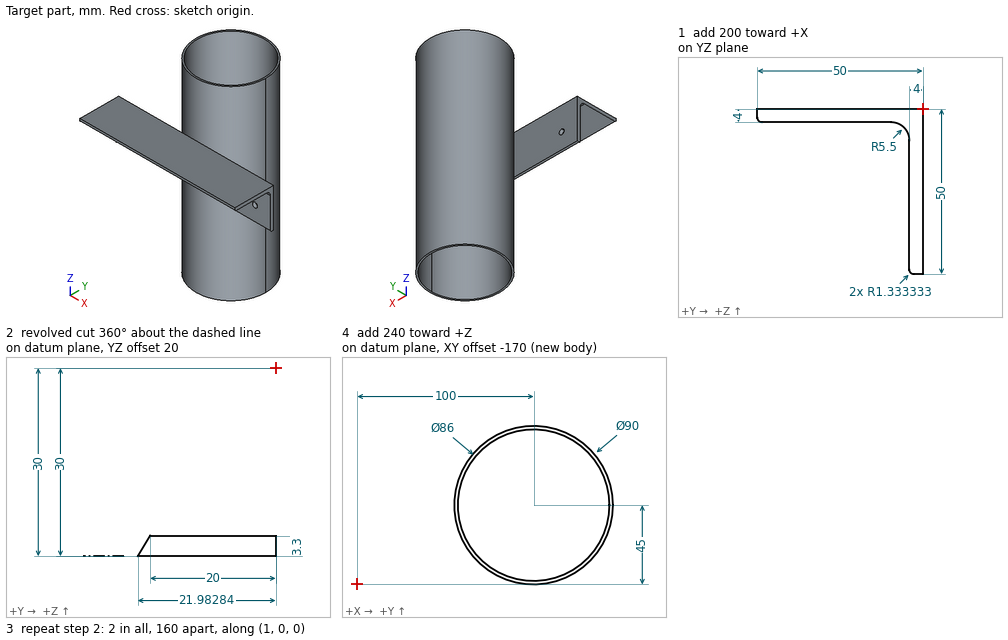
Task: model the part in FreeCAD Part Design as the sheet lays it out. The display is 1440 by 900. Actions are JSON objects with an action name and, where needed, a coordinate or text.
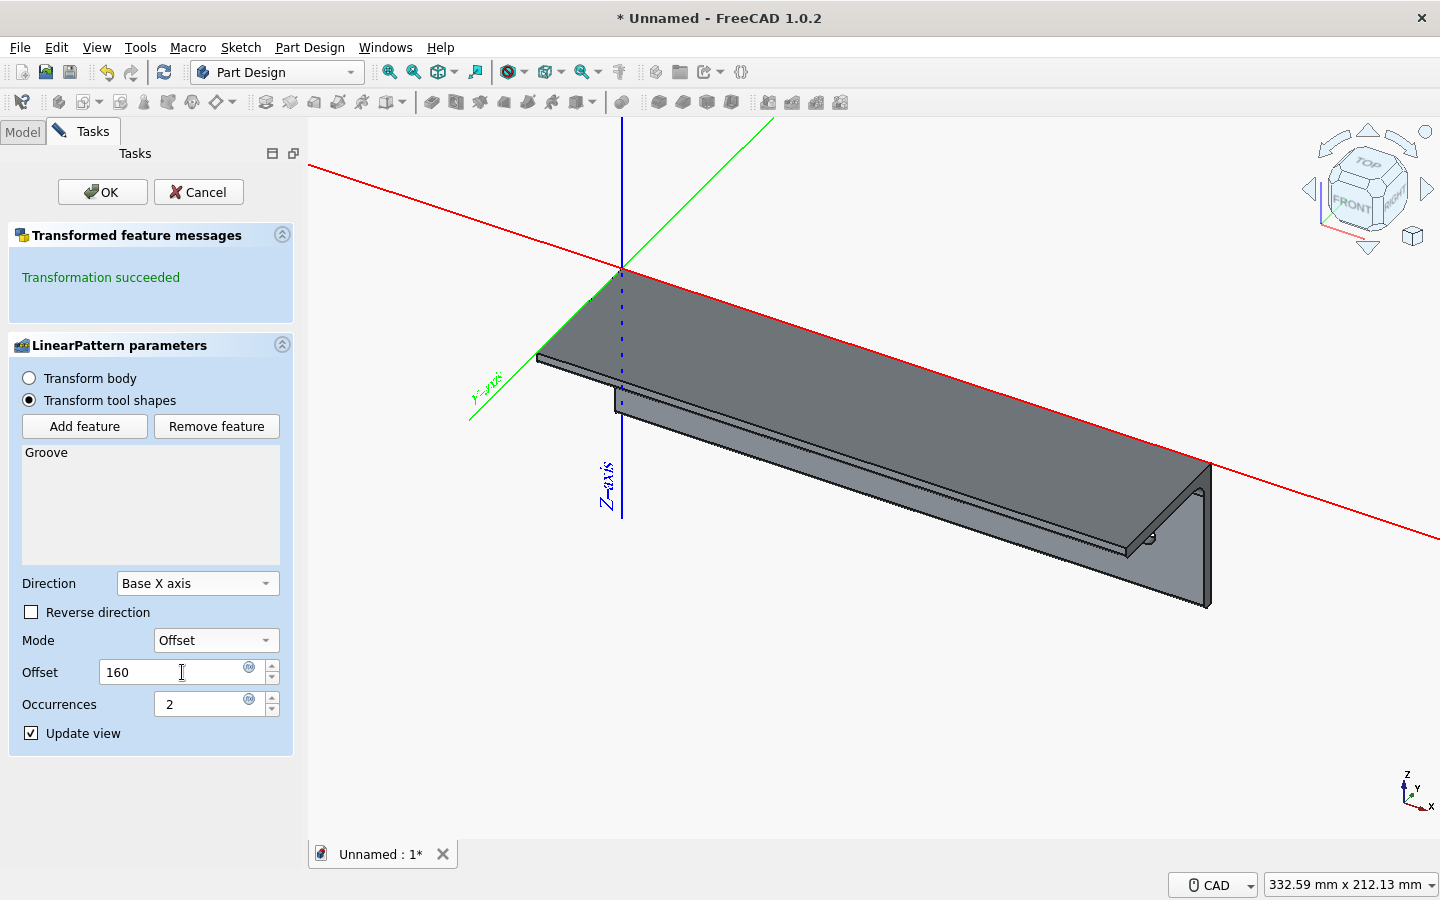
{"action": "triple_click", "coordinate": [209, 704]}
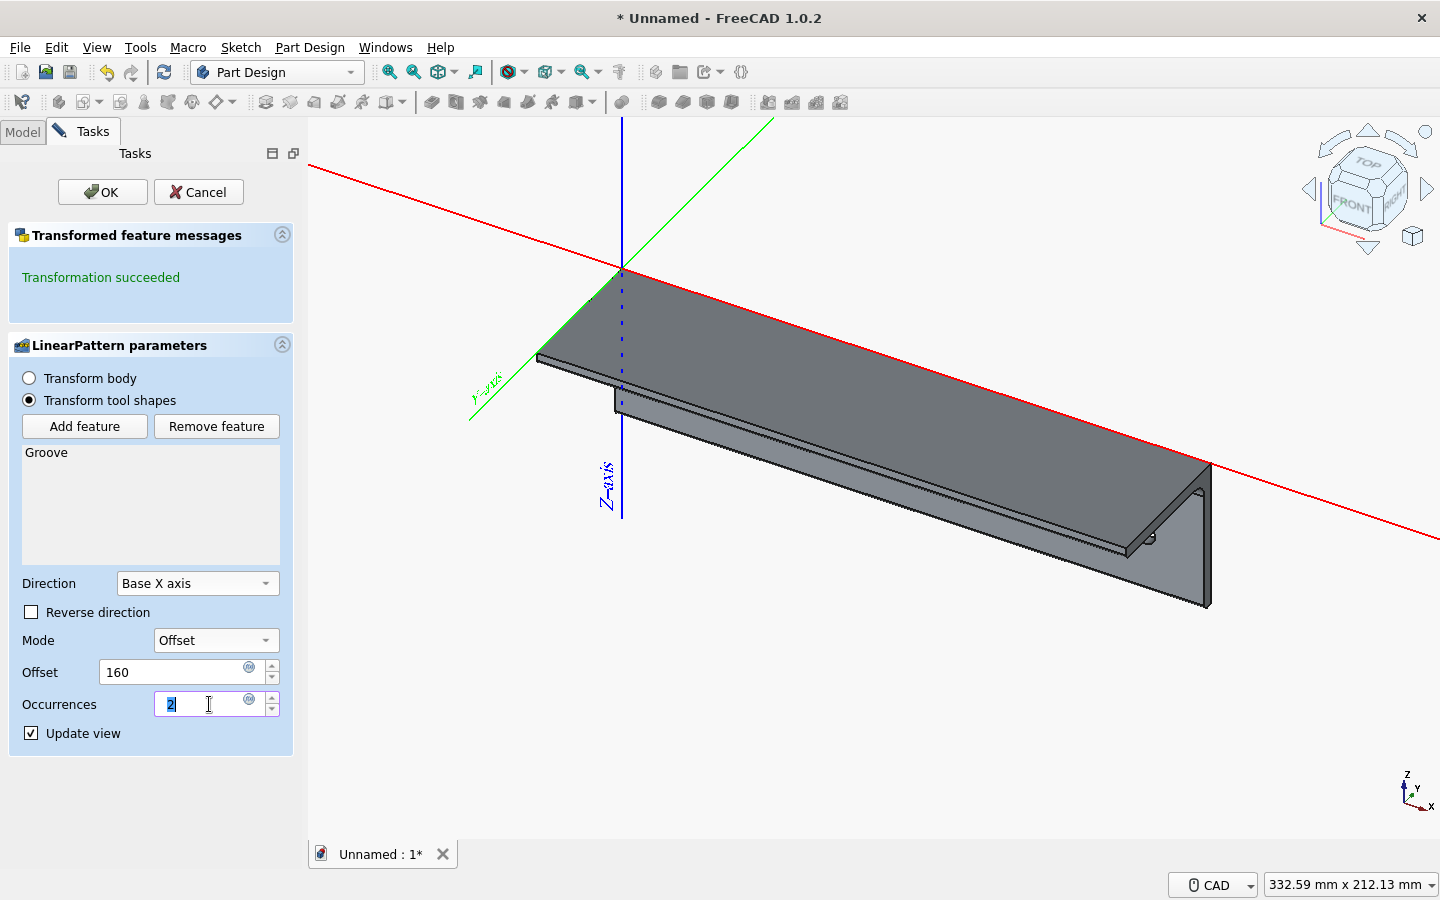
{"action": "type", "text": "2"}
{"action": "key", "text": "Tab"}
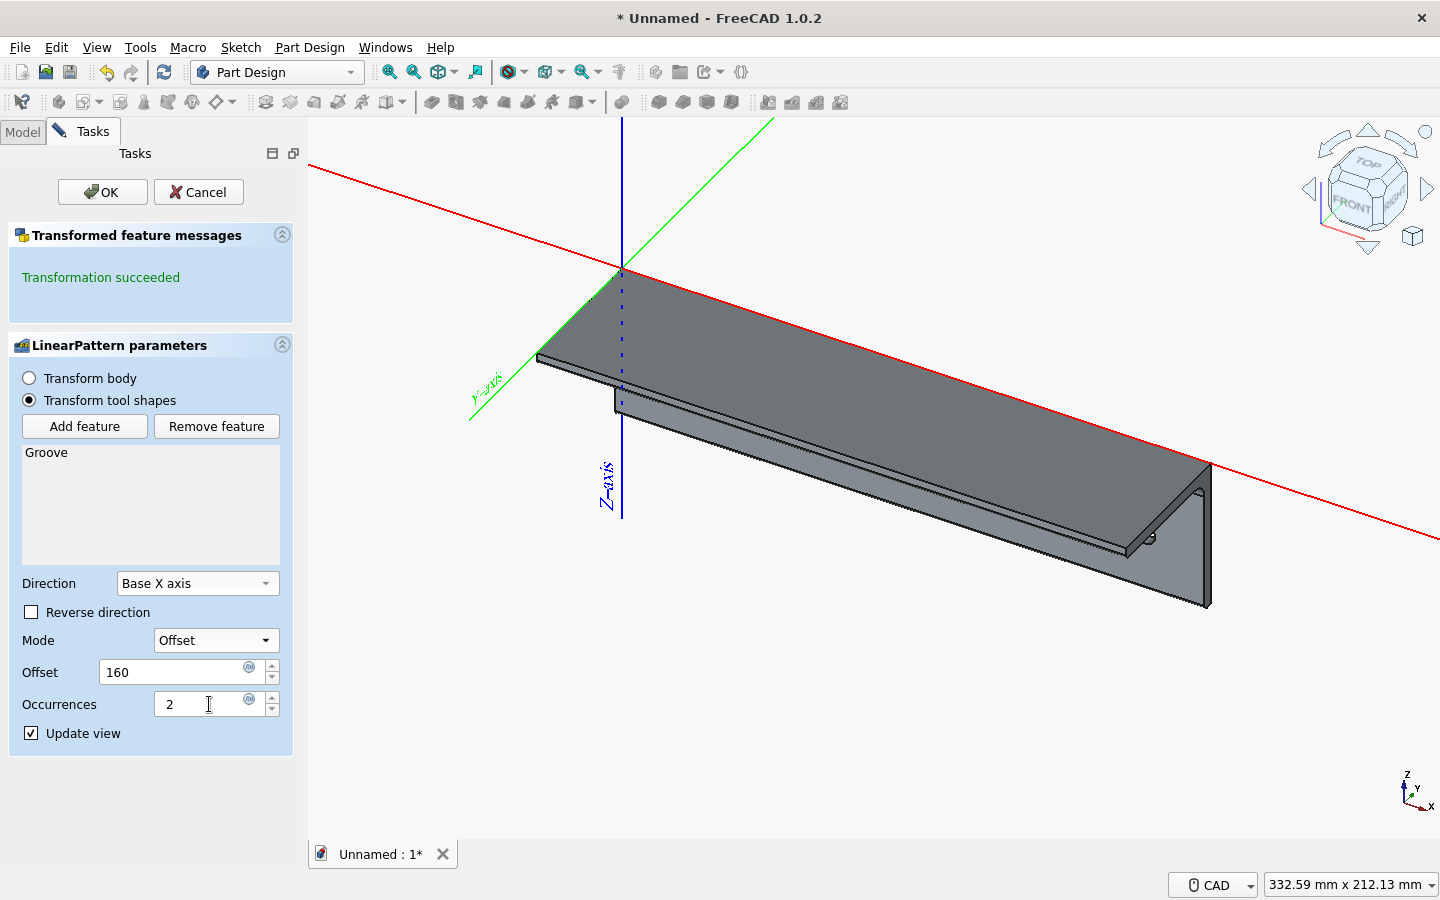
{"action": "left_click", "coordinate": [103, 192]}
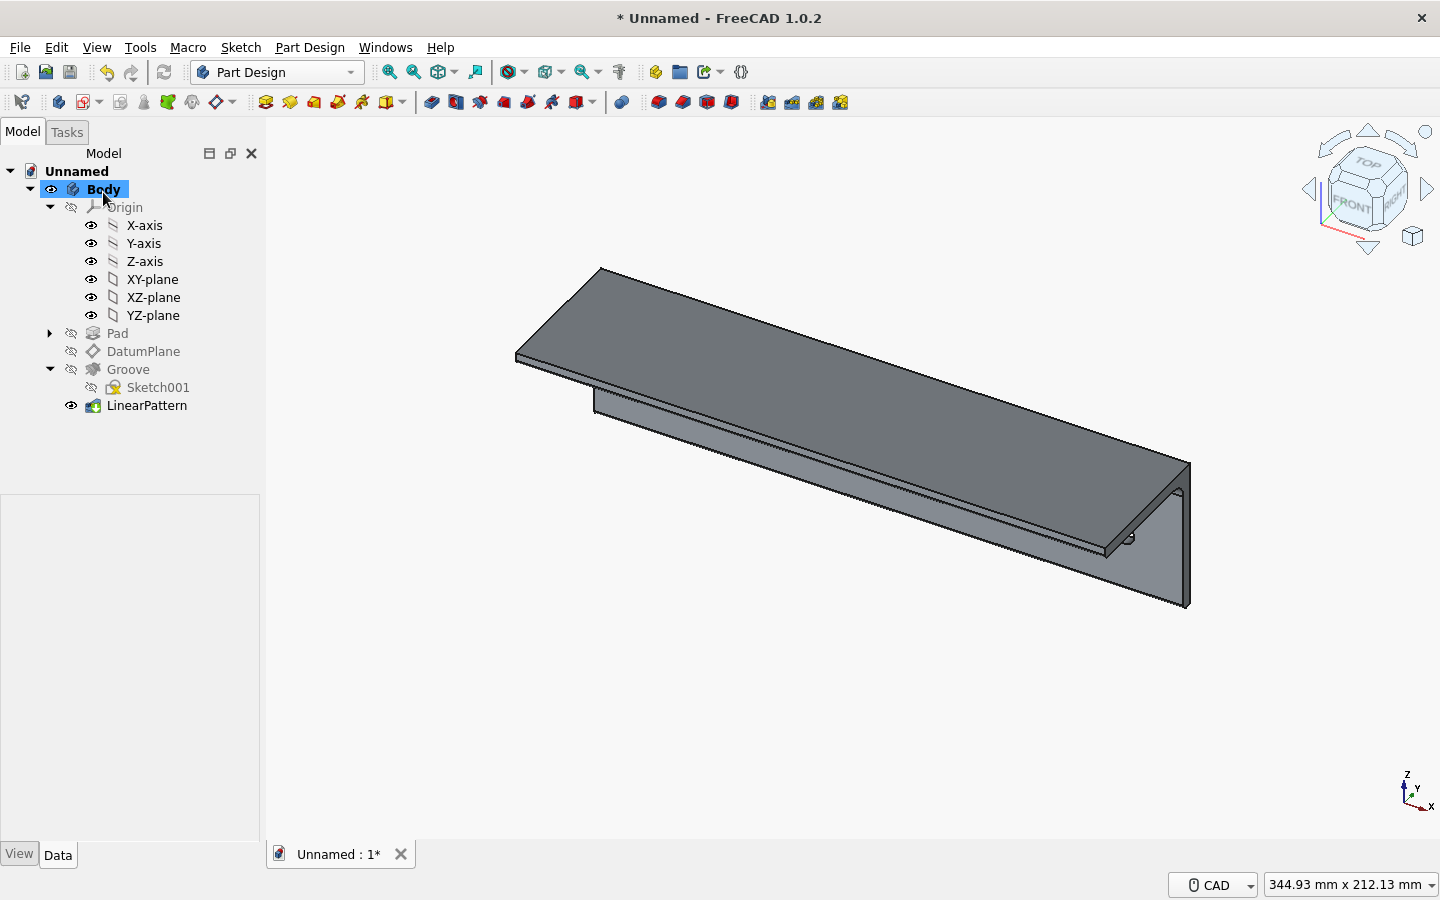
{"action": "left_click", "coordinate": [60, 102]}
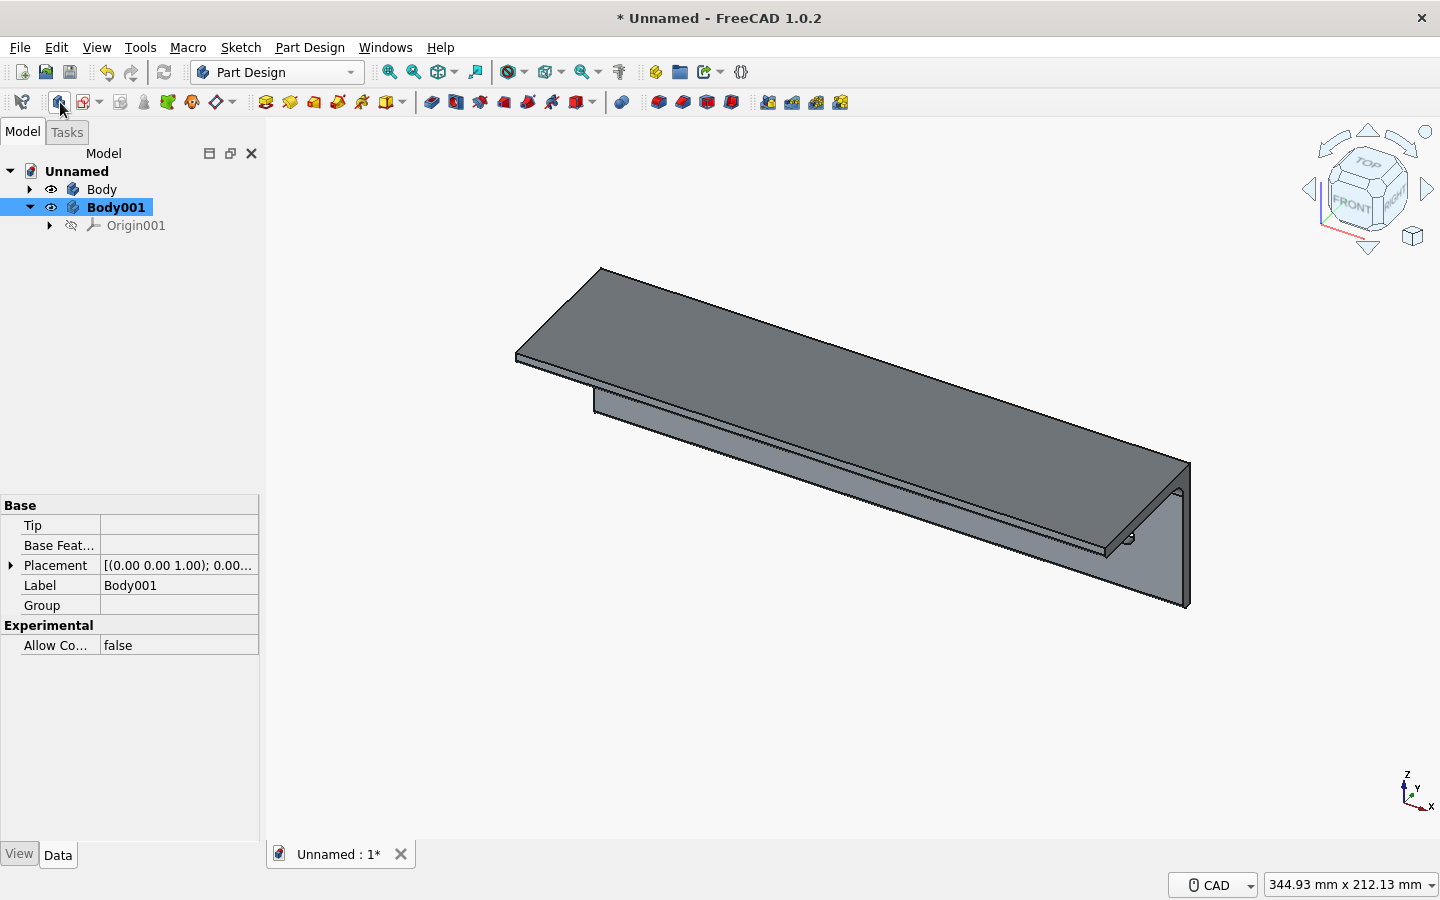
{"action": "left_click", "coordinate": [50, 225]}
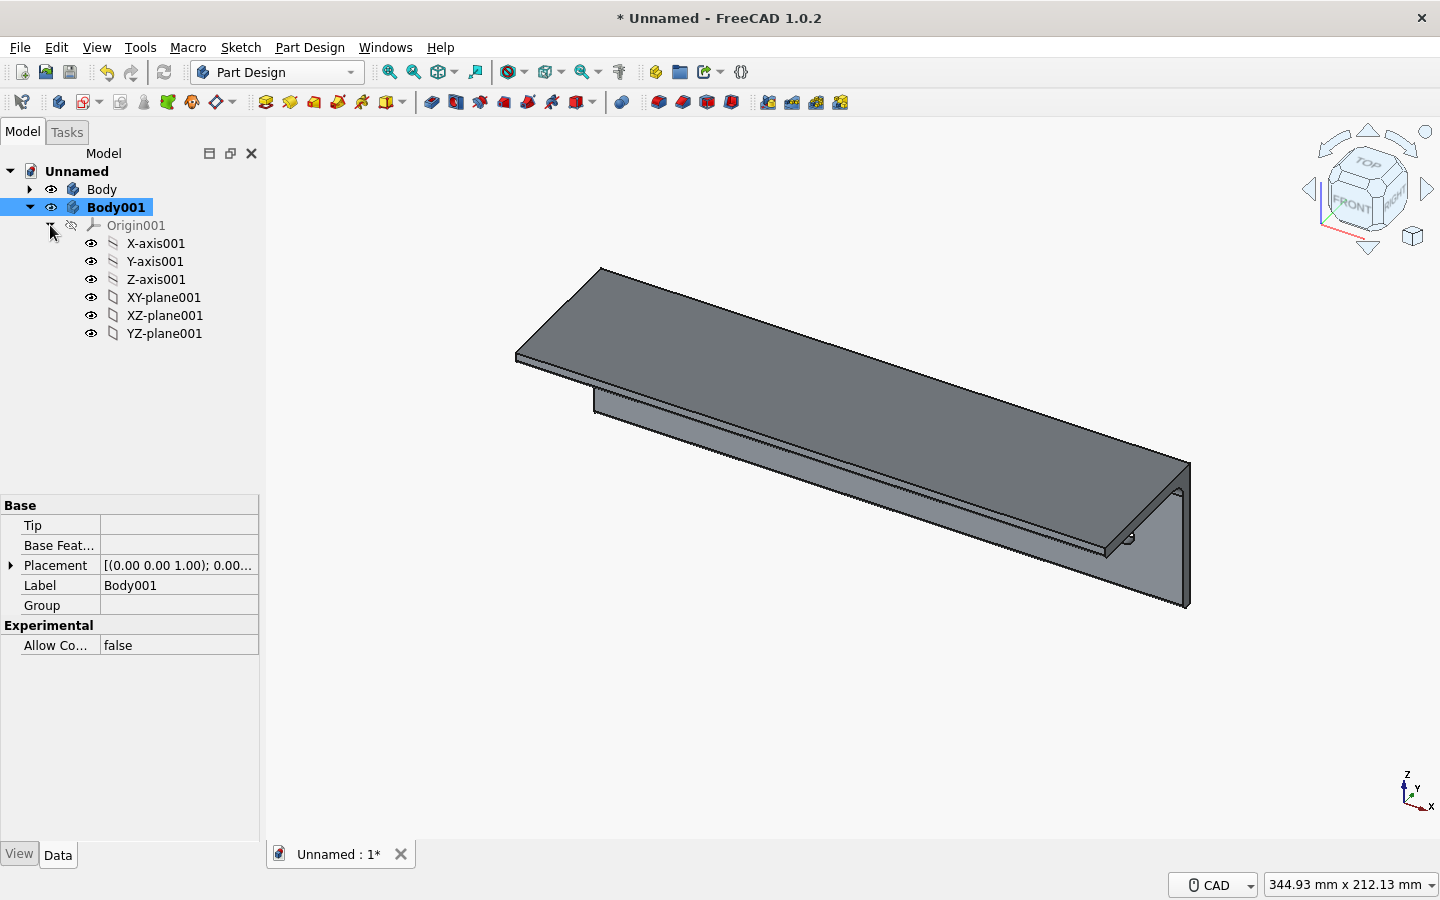
{"action": "left_click", "coordinate": [136, 297]}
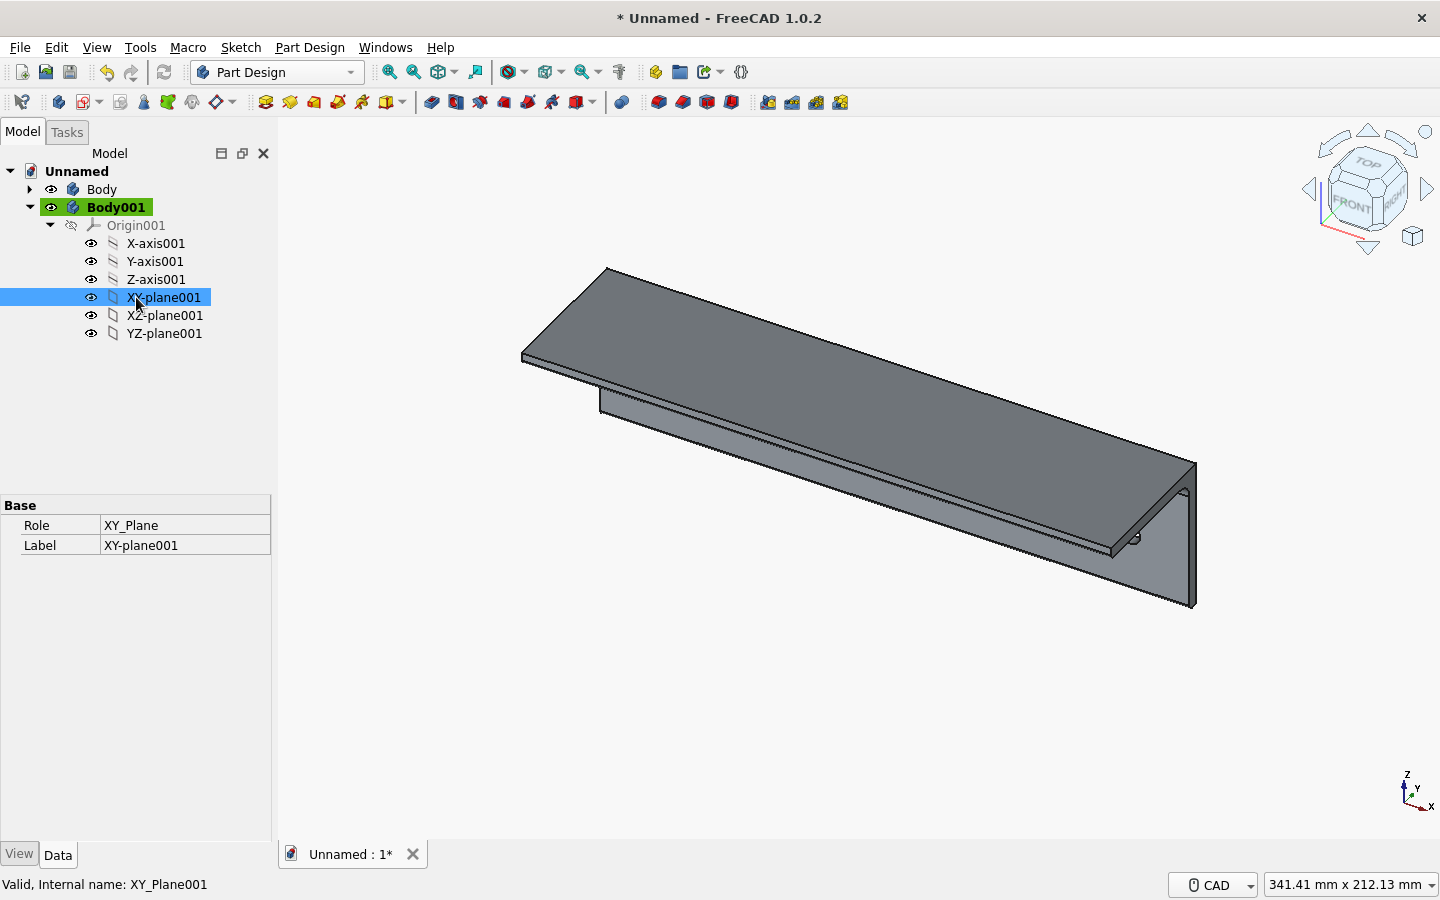
{"action": "left_click", "coordinate": [216, 102]}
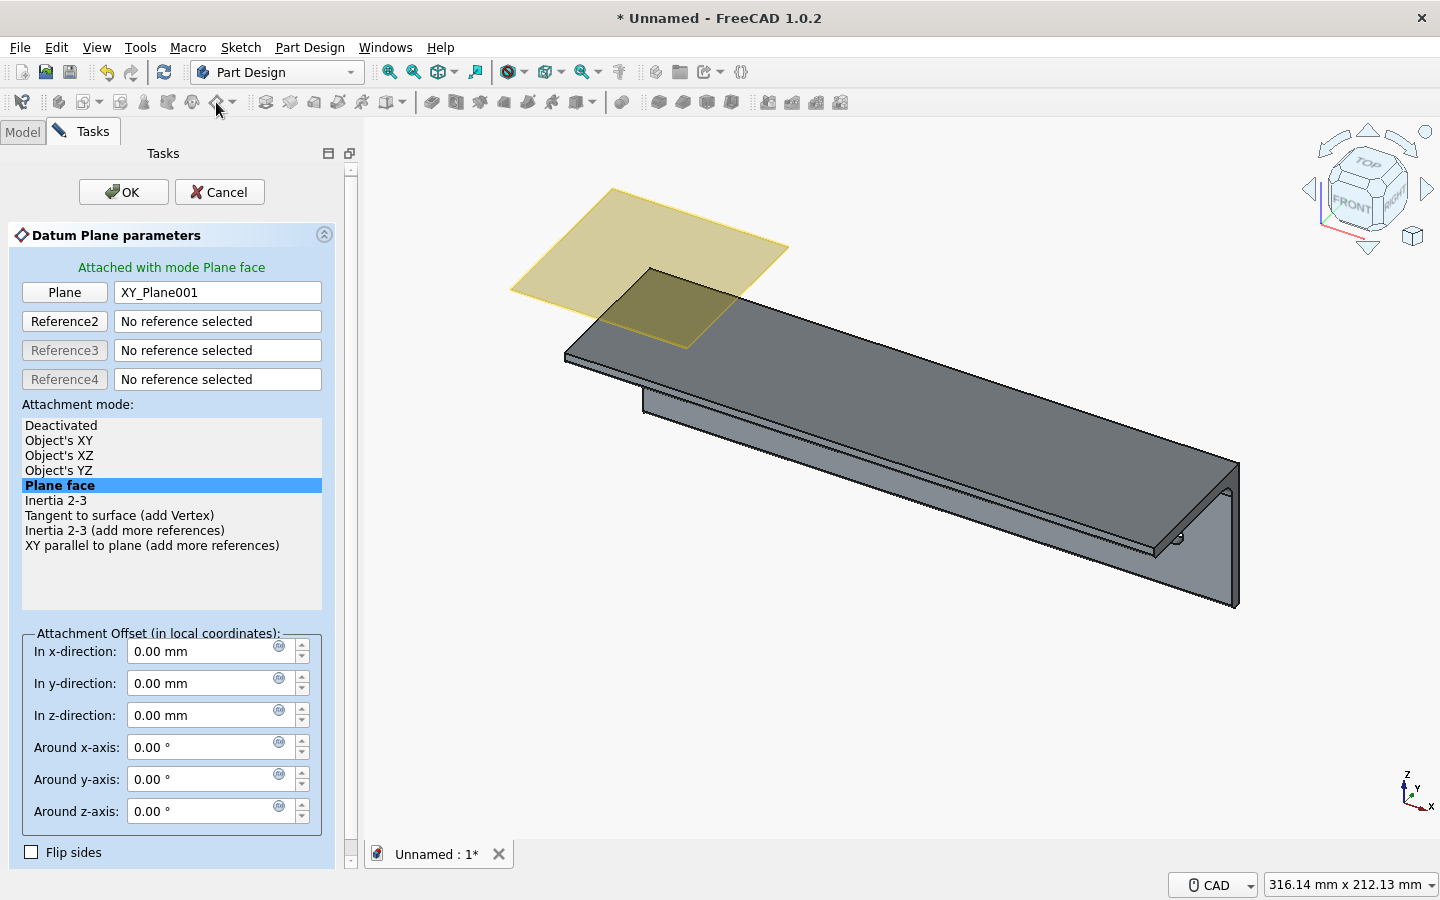
{"action": "triple_click", "coordinate": [210, 715]}